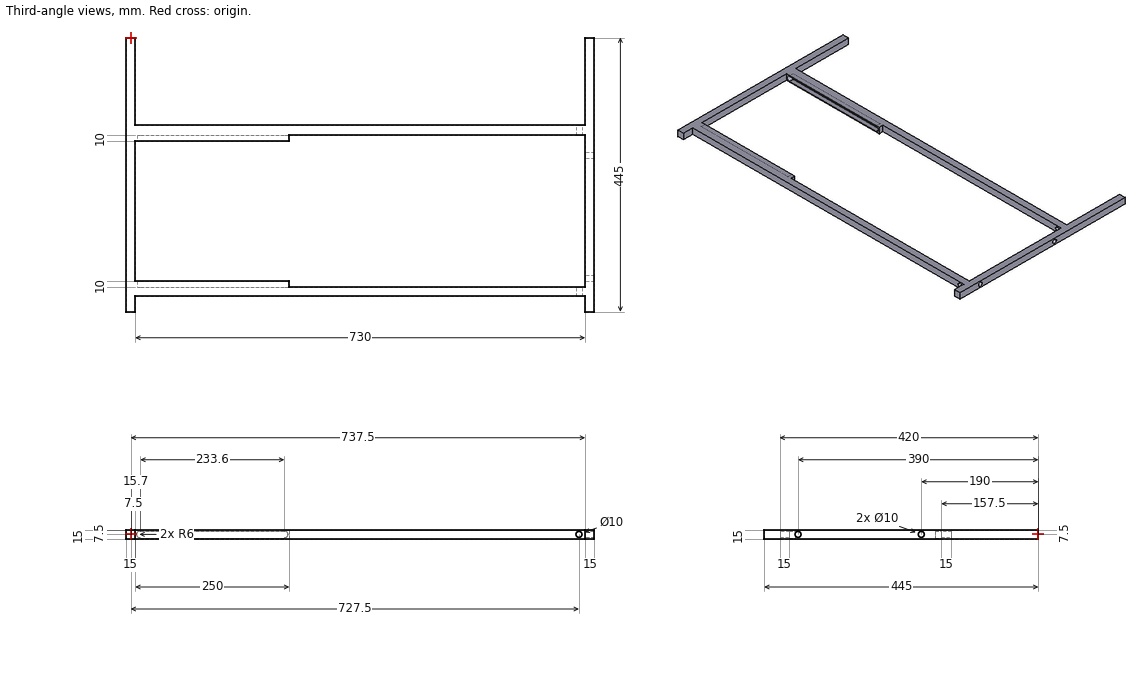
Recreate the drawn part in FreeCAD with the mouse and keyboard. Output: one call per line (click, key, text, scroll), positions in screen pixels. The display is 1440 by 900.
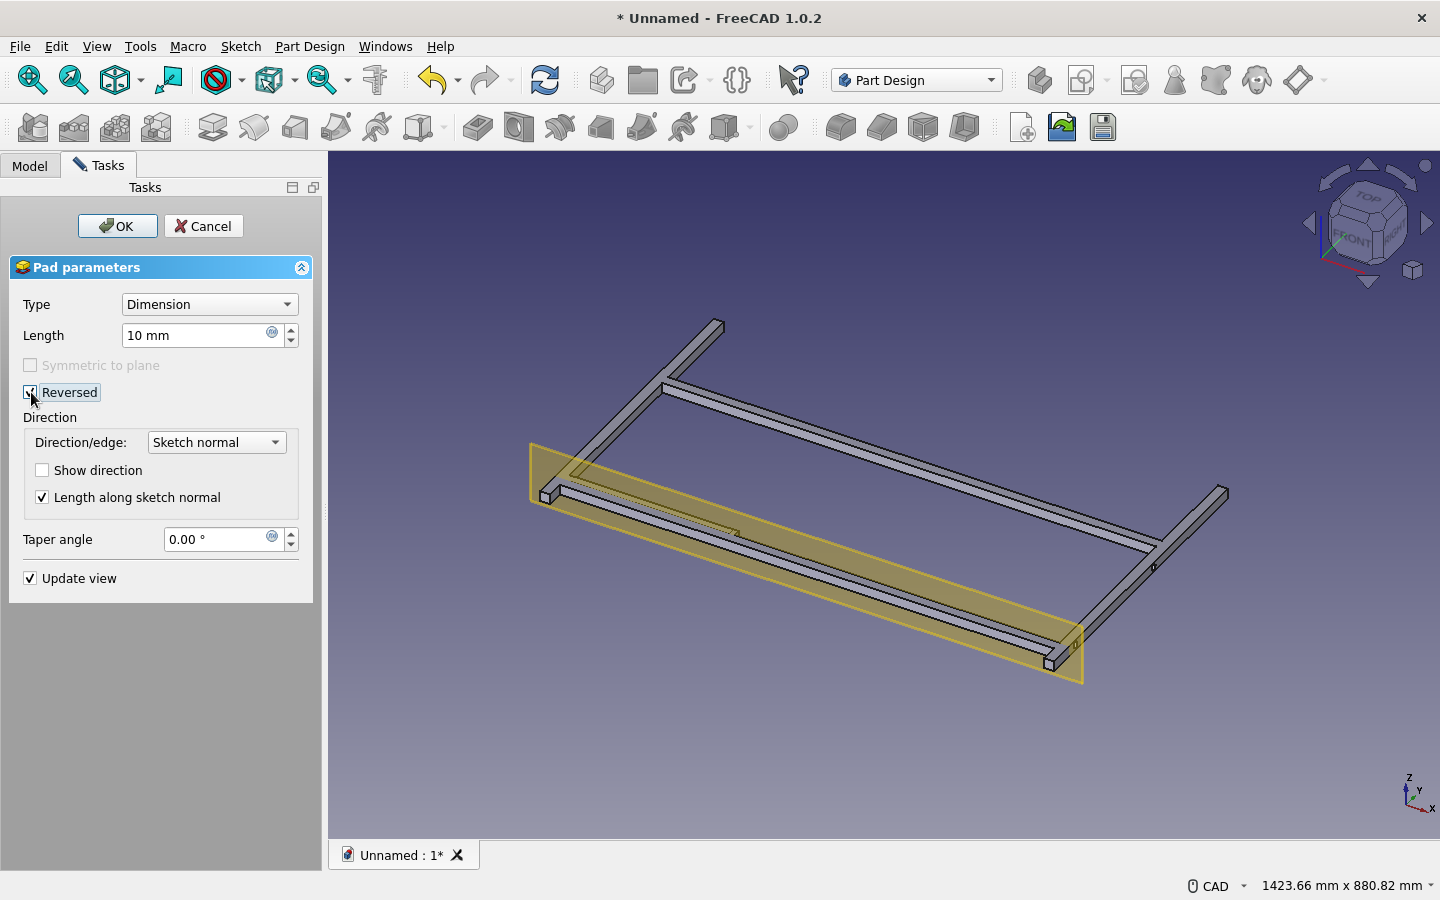
click(118, 226)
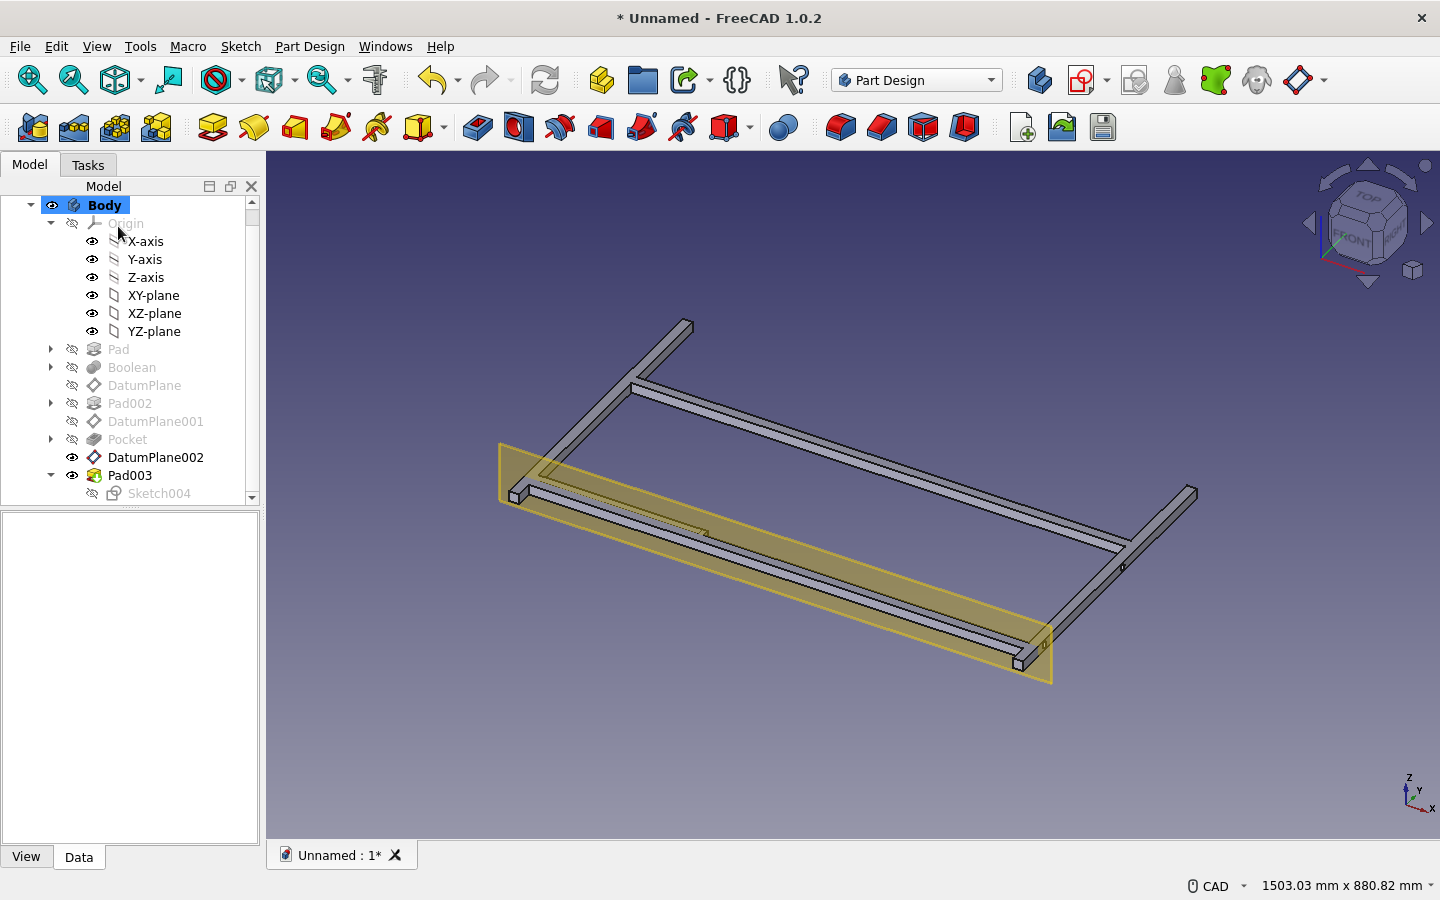
click(117, 457)
key(space)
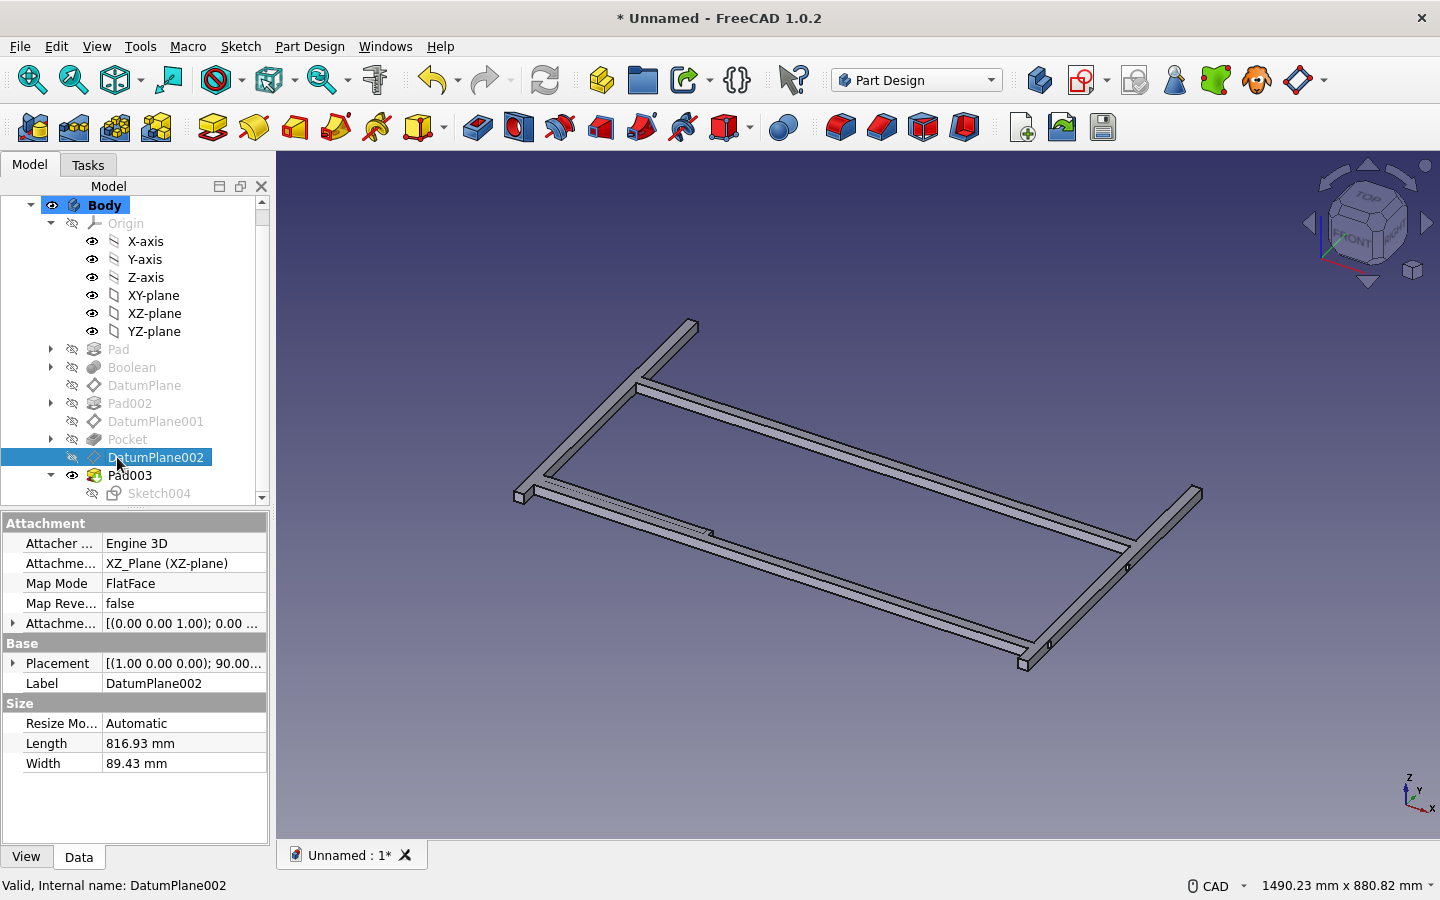
click(137, 313)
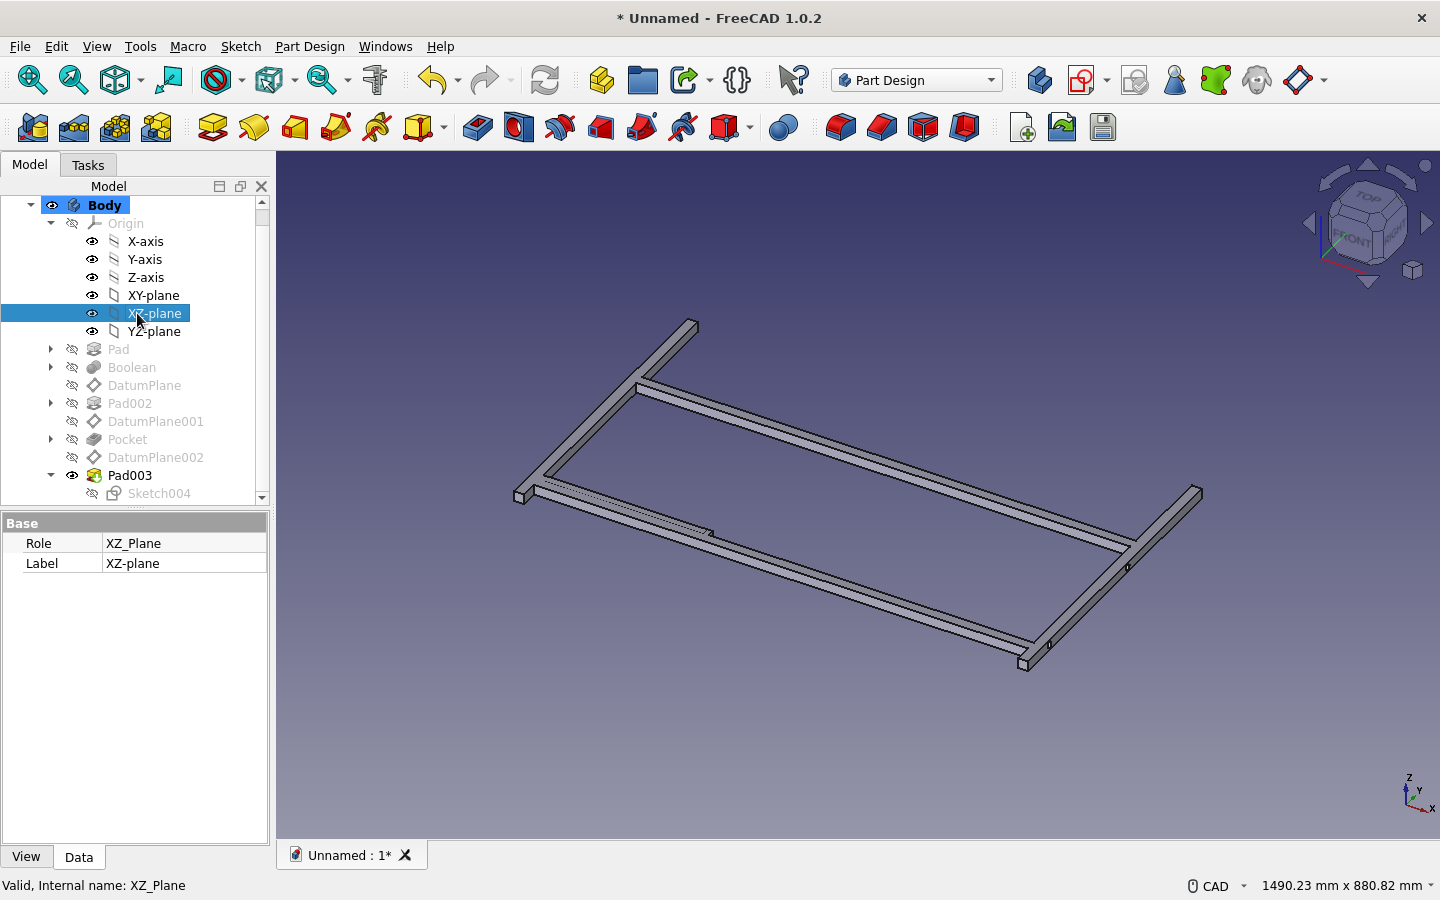
click(1298, 80)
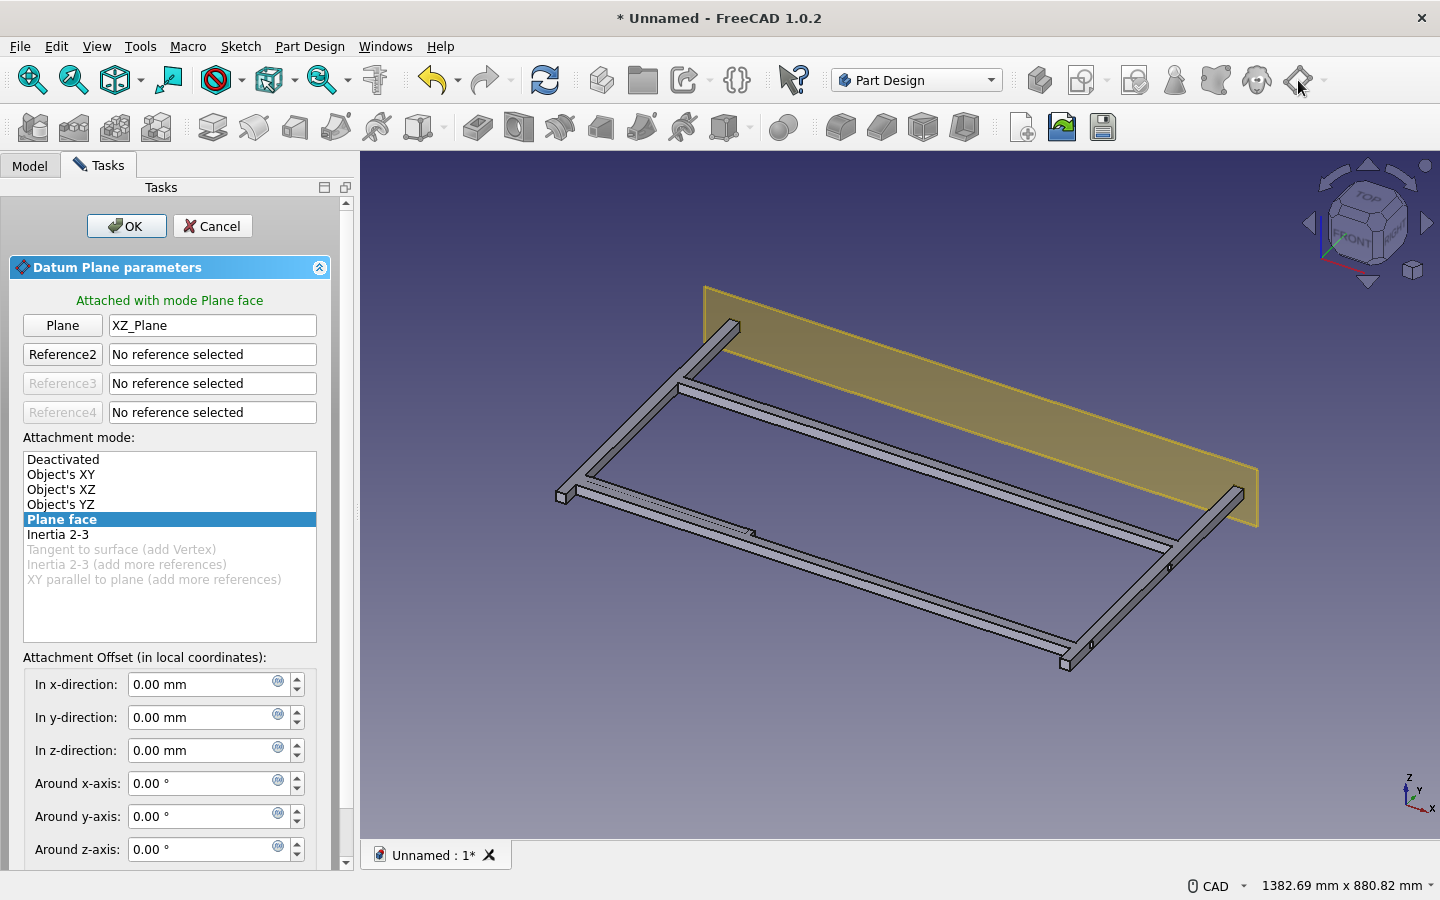
triple_click(210, 750)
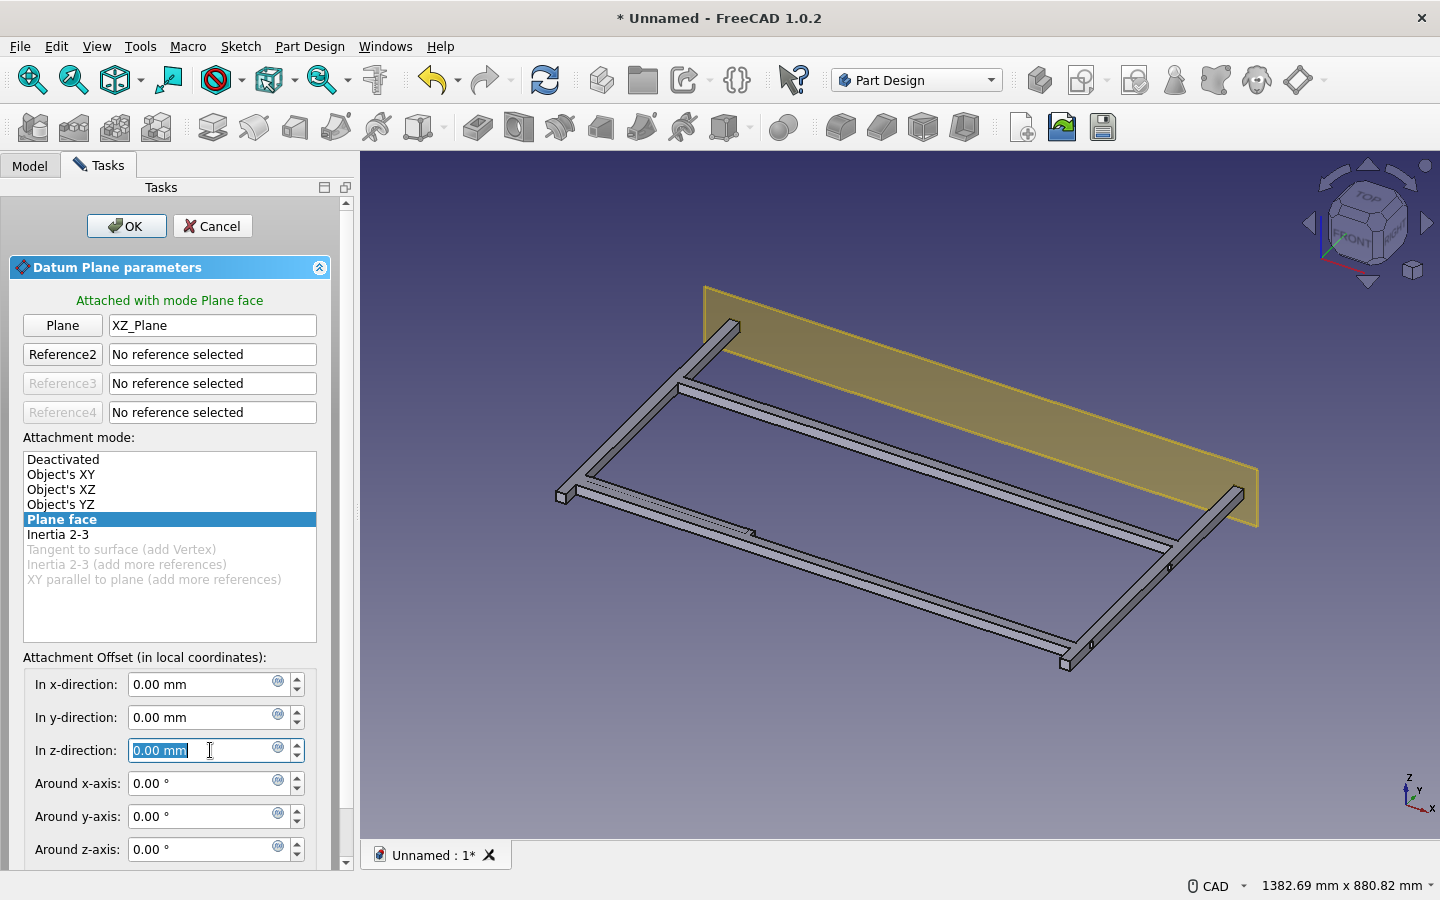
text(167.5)
key(Tab)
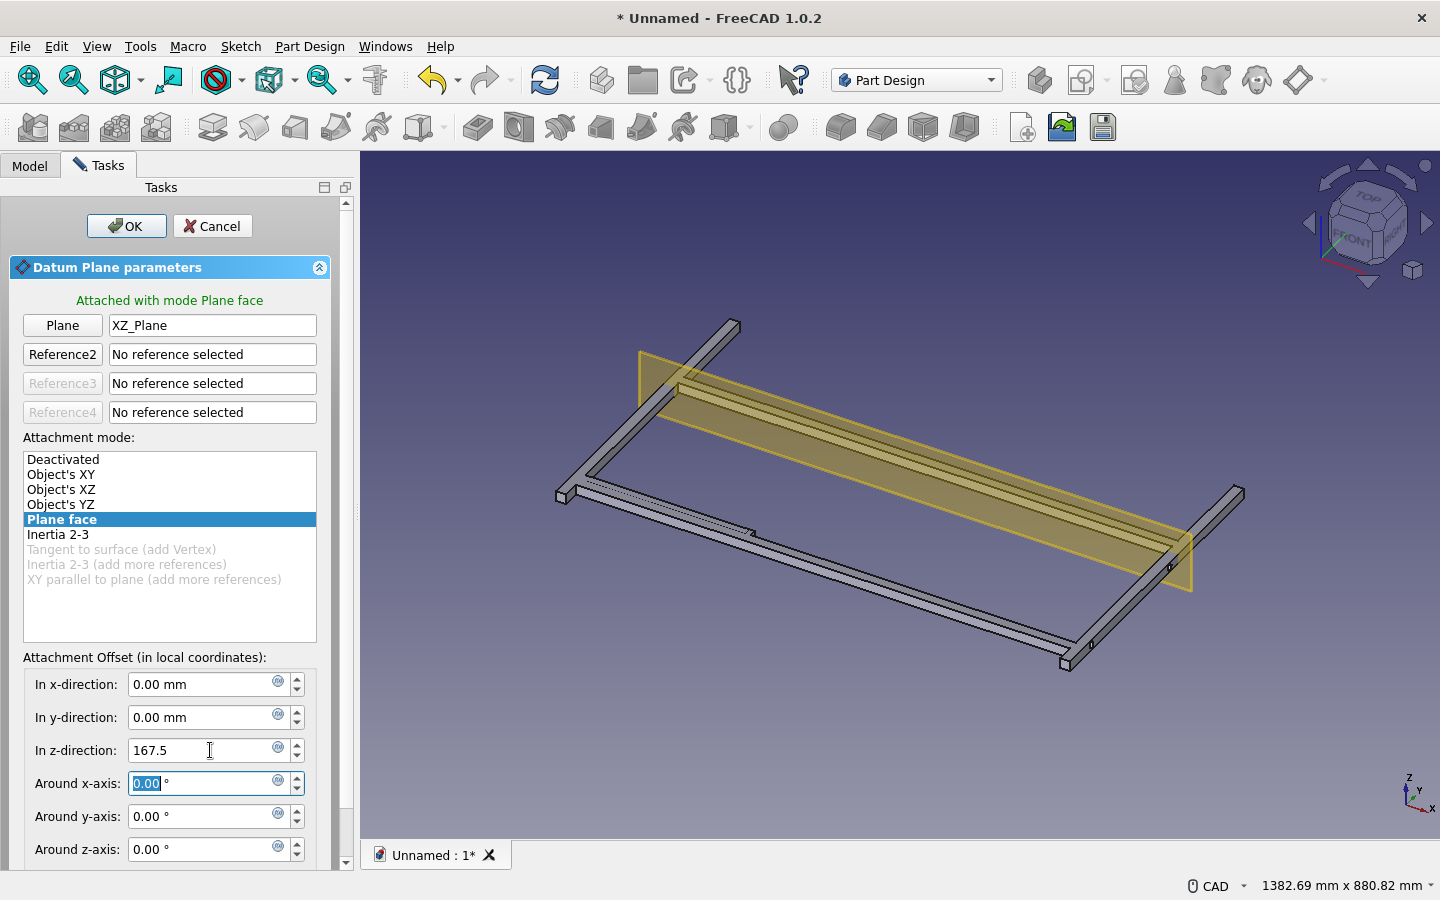
click(127, 226)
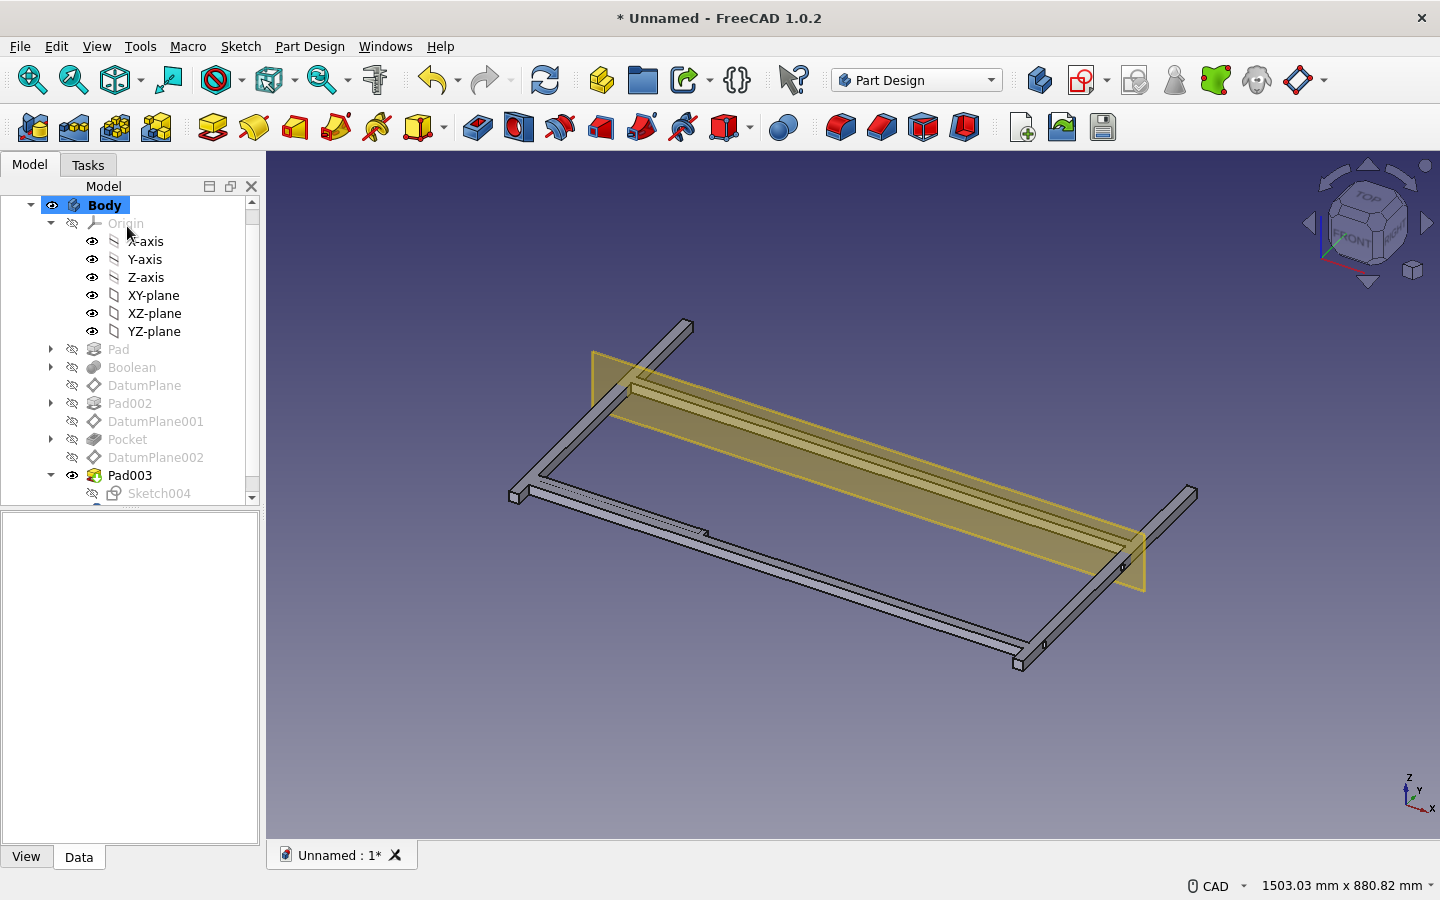
scroll(121, 345, down, 3)